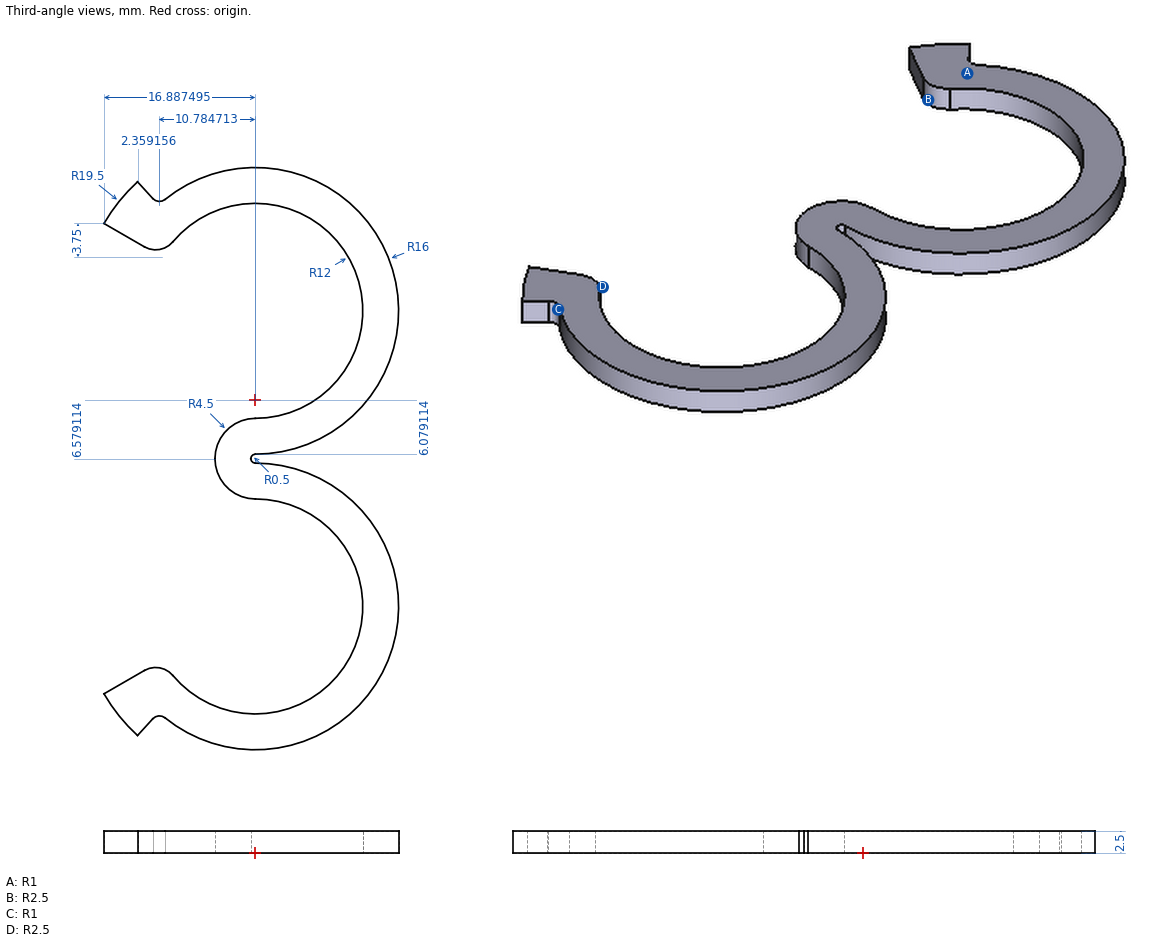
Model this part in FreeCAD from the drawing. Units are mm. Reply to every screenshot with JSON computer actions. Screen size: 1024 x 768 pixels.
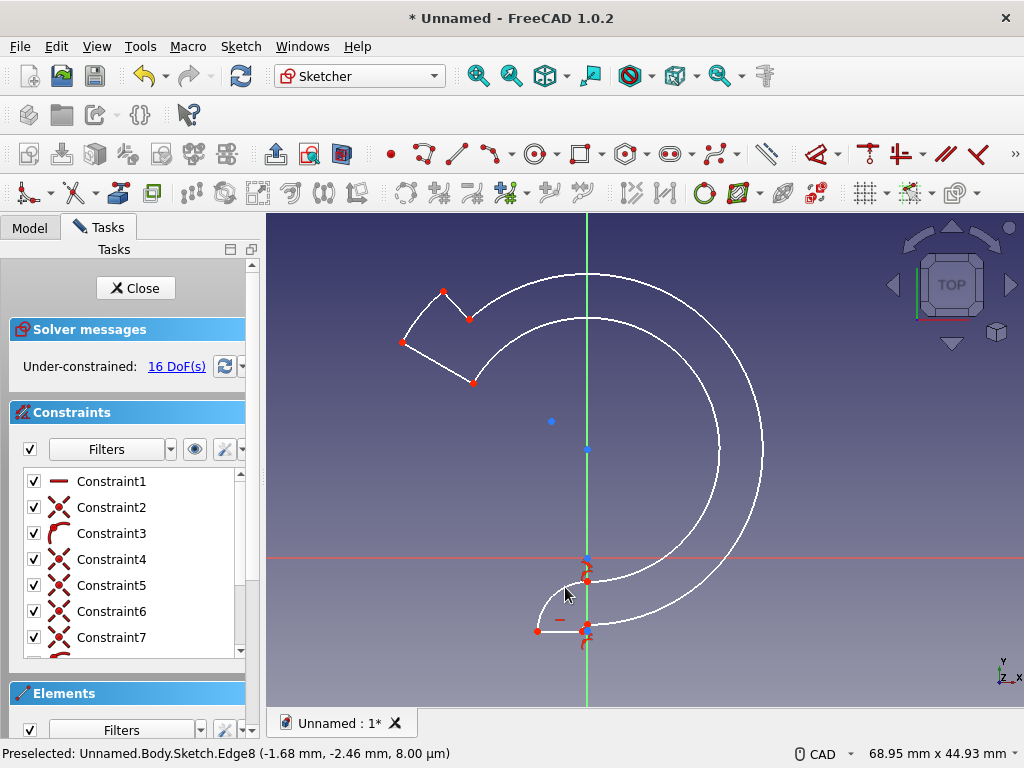
{"action": "left_click", "coordinate": [749, 519]}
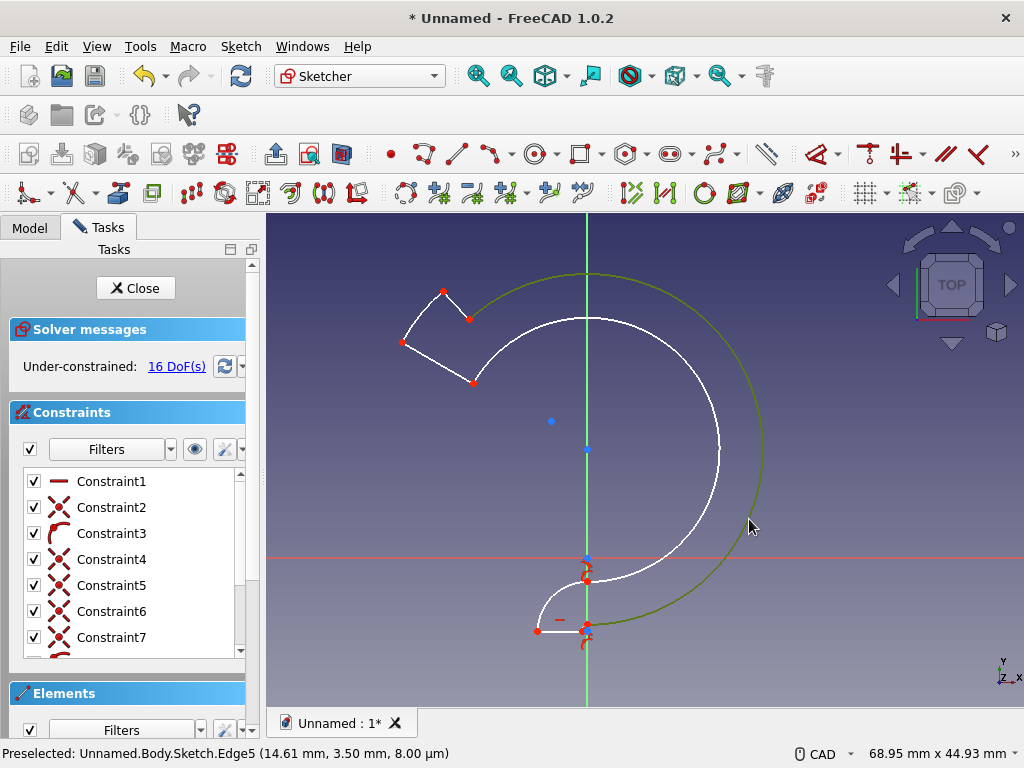
{"action": "left_click", "coordinate": [429, 305]}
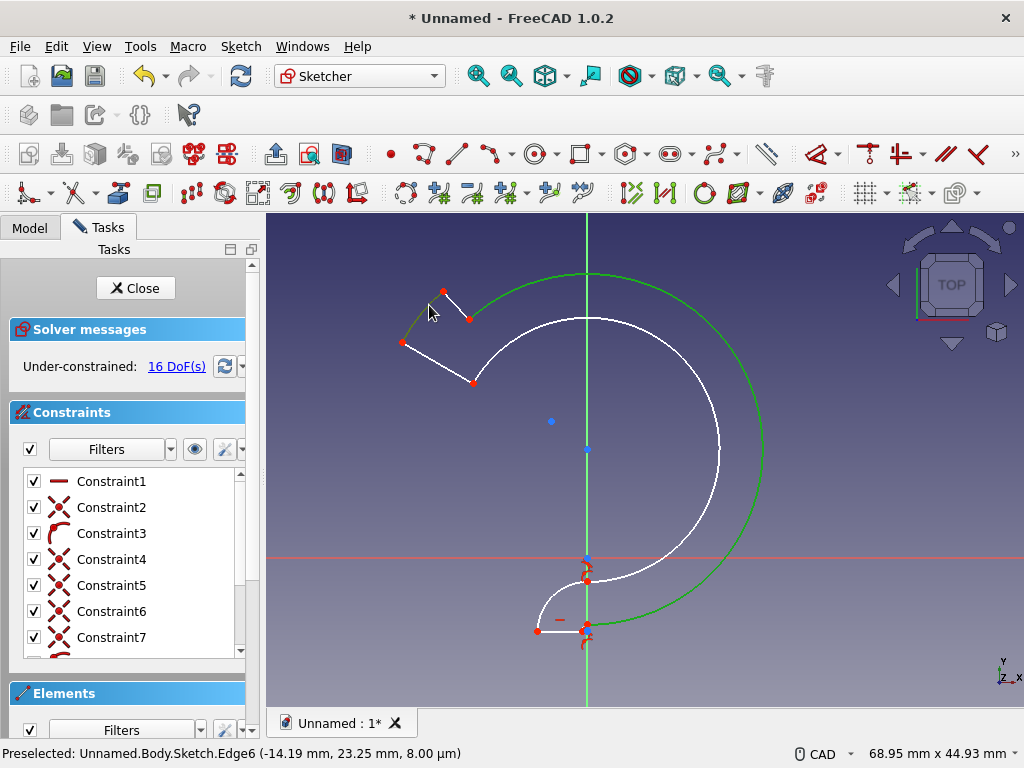
{"action": "left_click", "coordinate": [868, 154]}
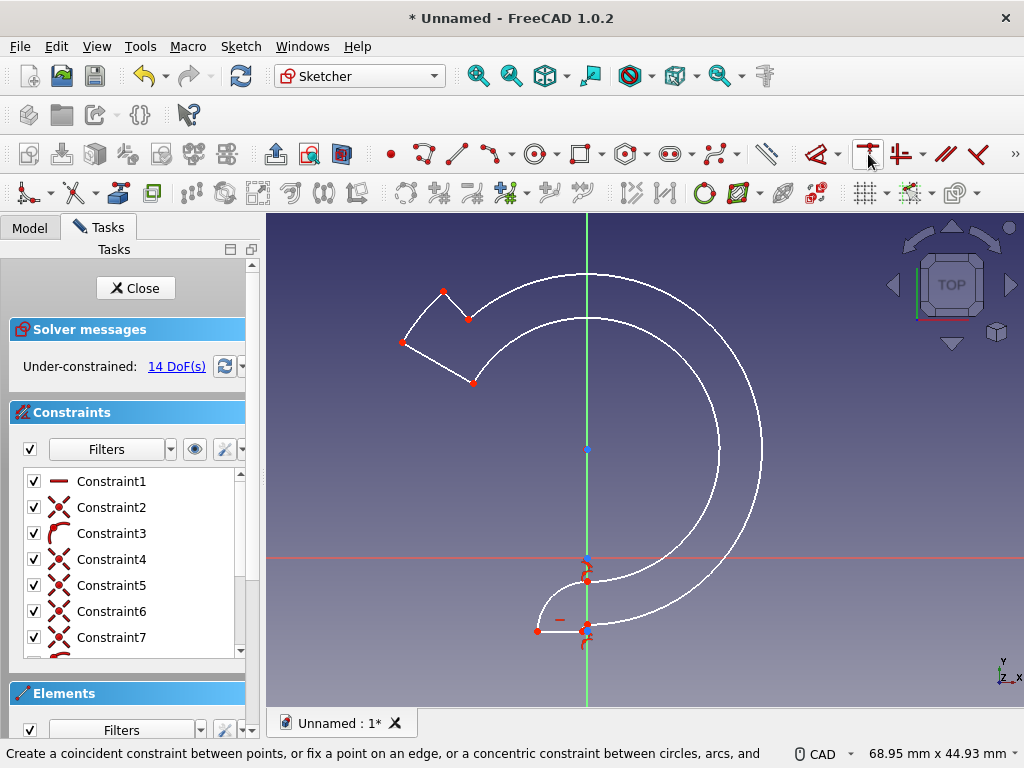
{"action": "left_click", "coordinate": [748, 518]}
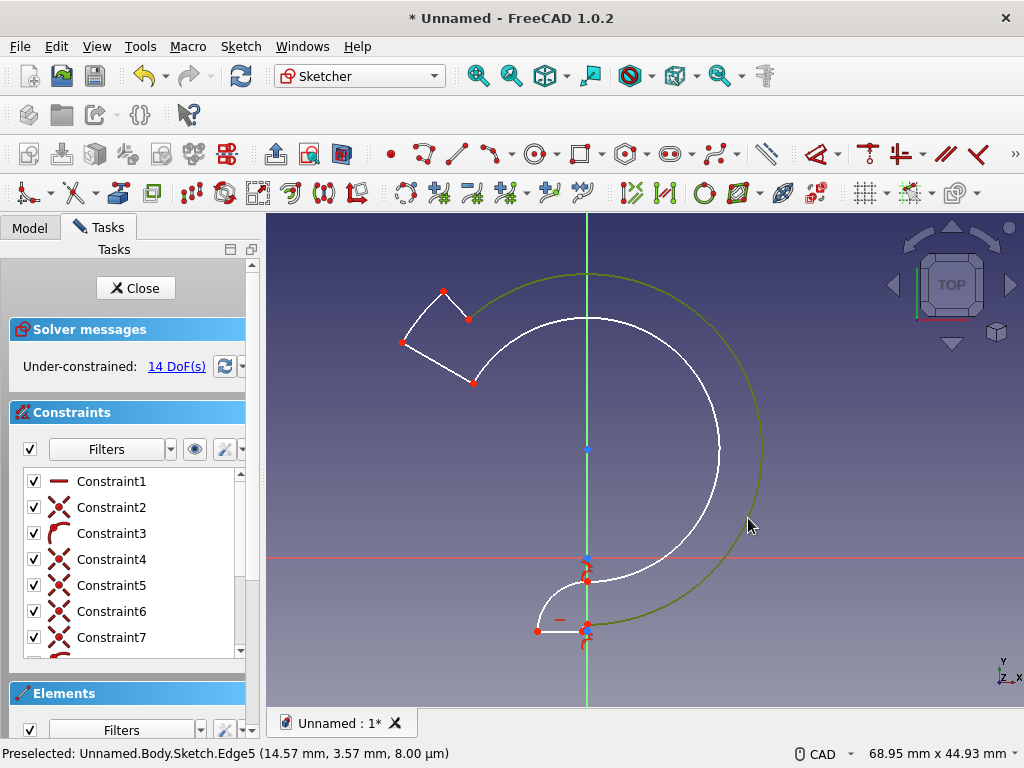
{"action": "left_click", "coordinate": [713, 491]}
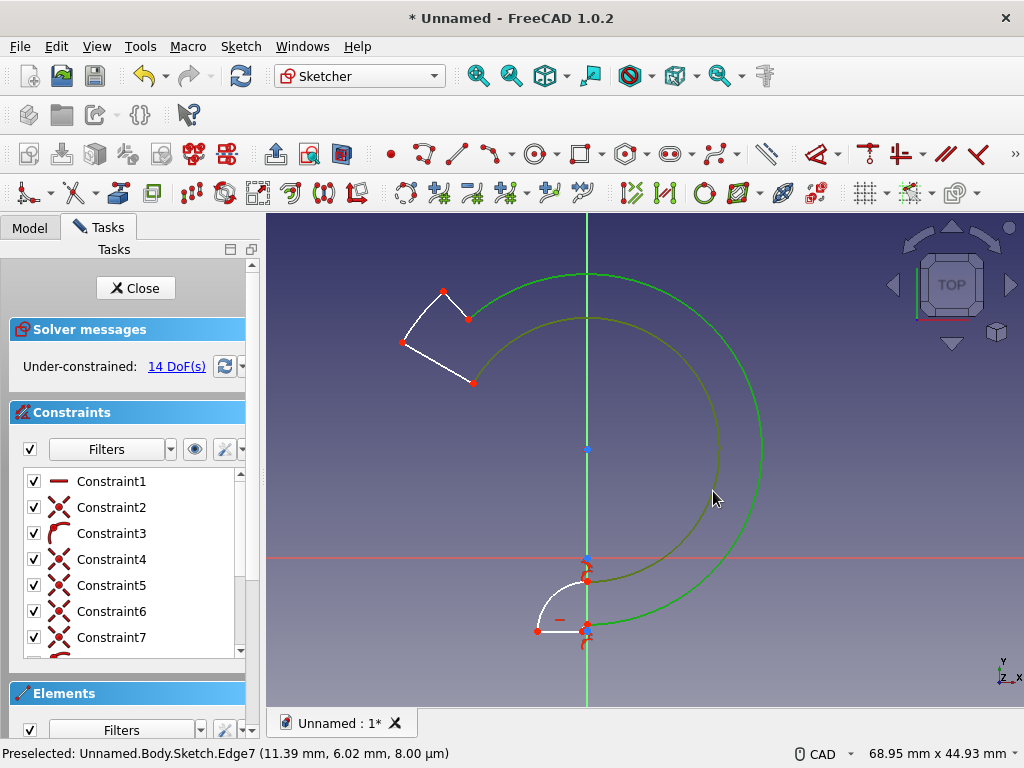
{"action": "left_click", "coordinate": [868, 154]}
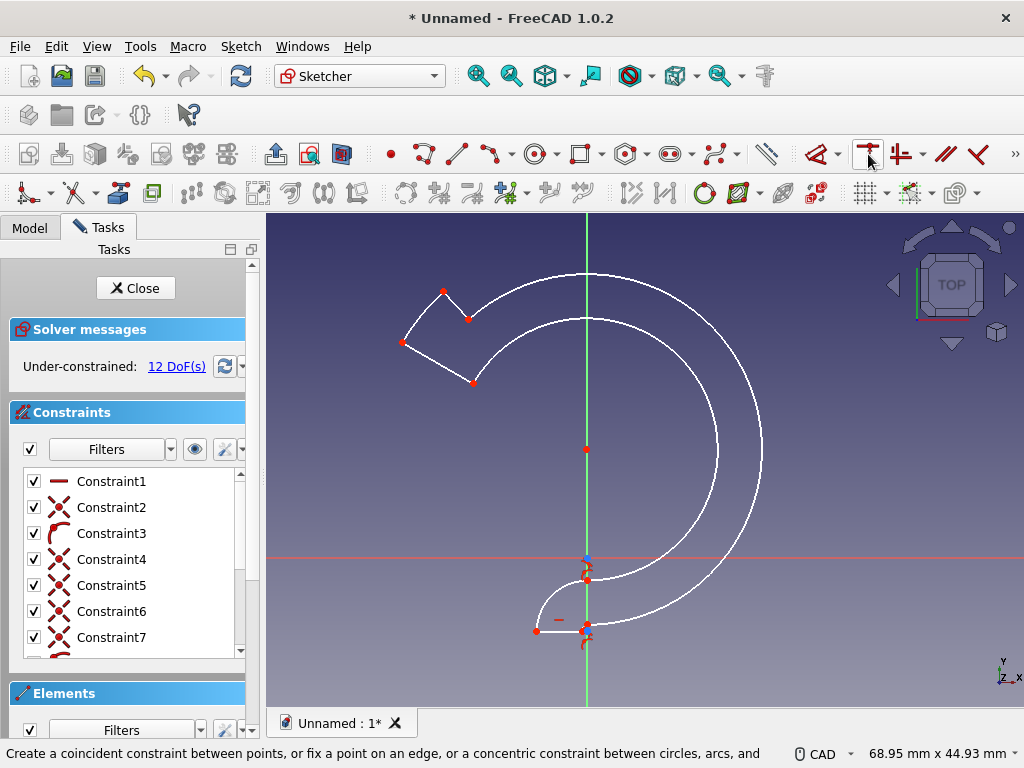
{"action": "left_click", "coordinate": [587, 449]}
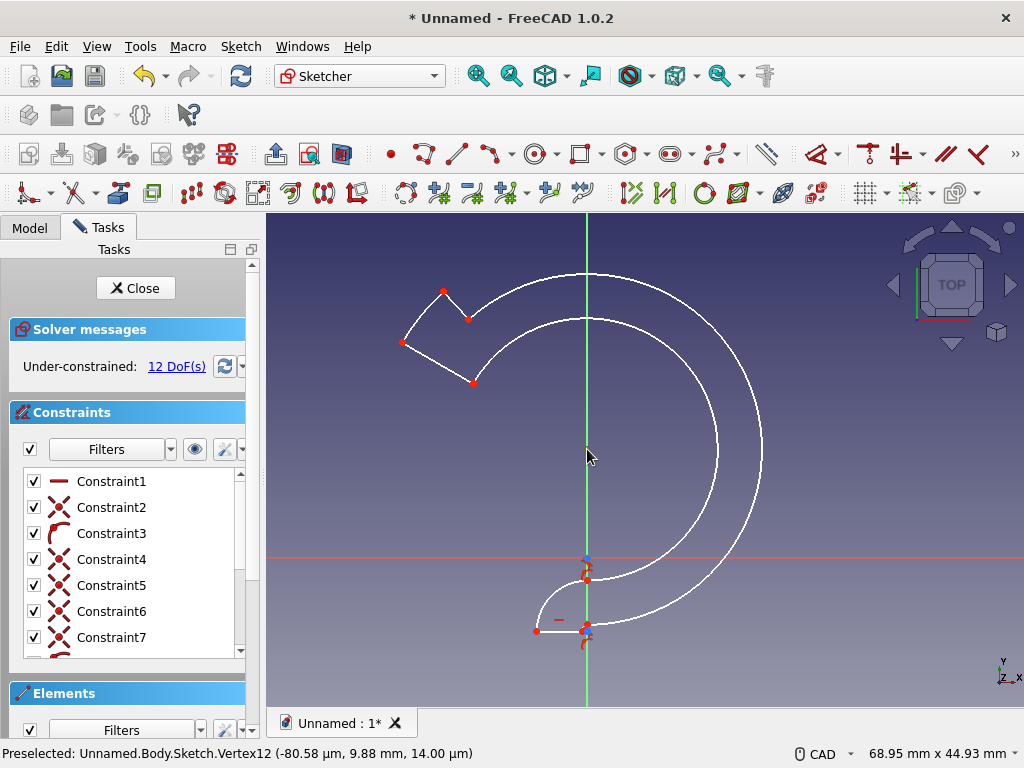
{"action": "left_click", "coordinate": [587, 523]}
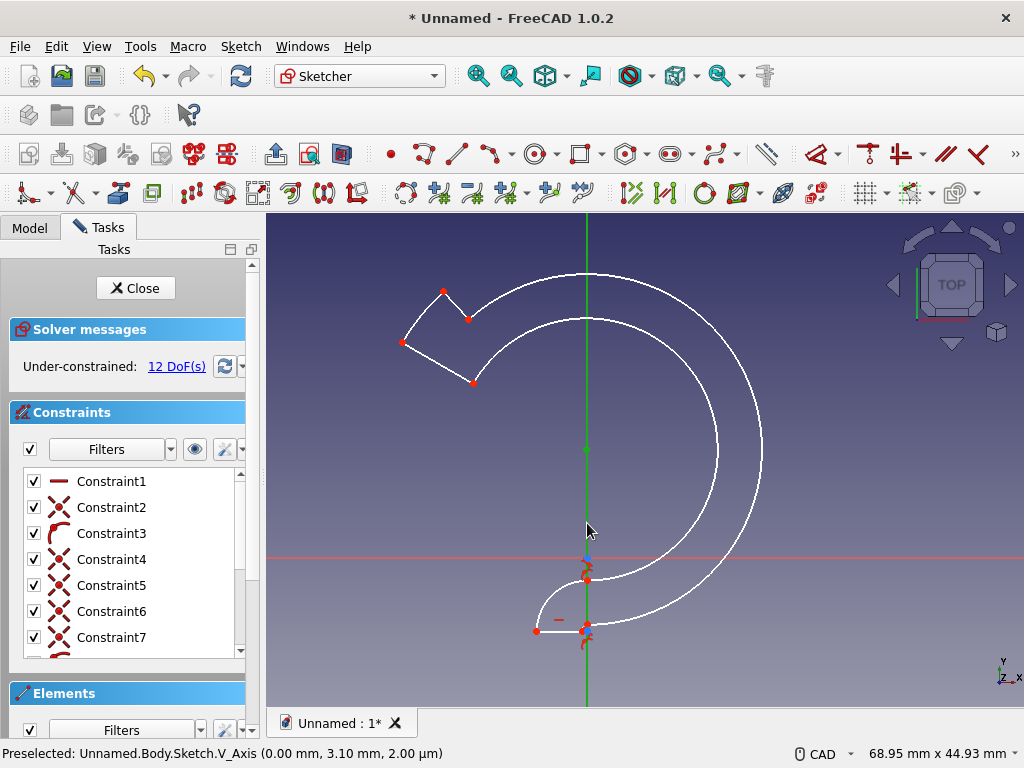
{"action": "left_click", "coordinate": [868, 154]}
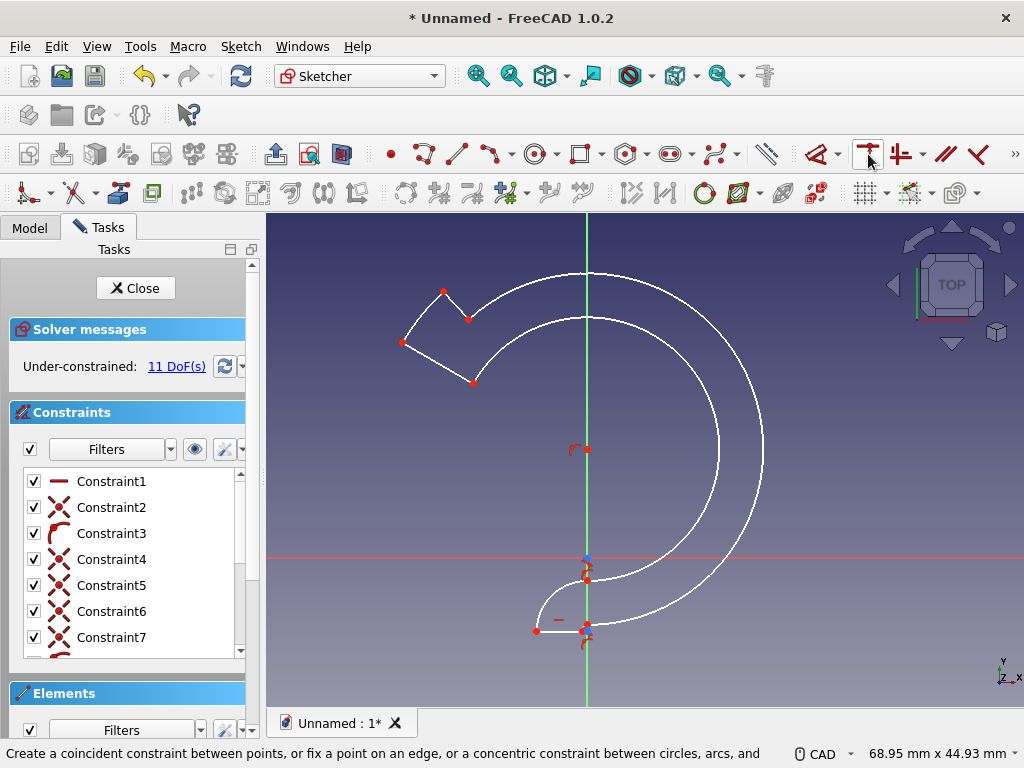
{"action": "scroll", "coordinate": [583, 627], "scroll_direction": "up", "scroll_amount": 10}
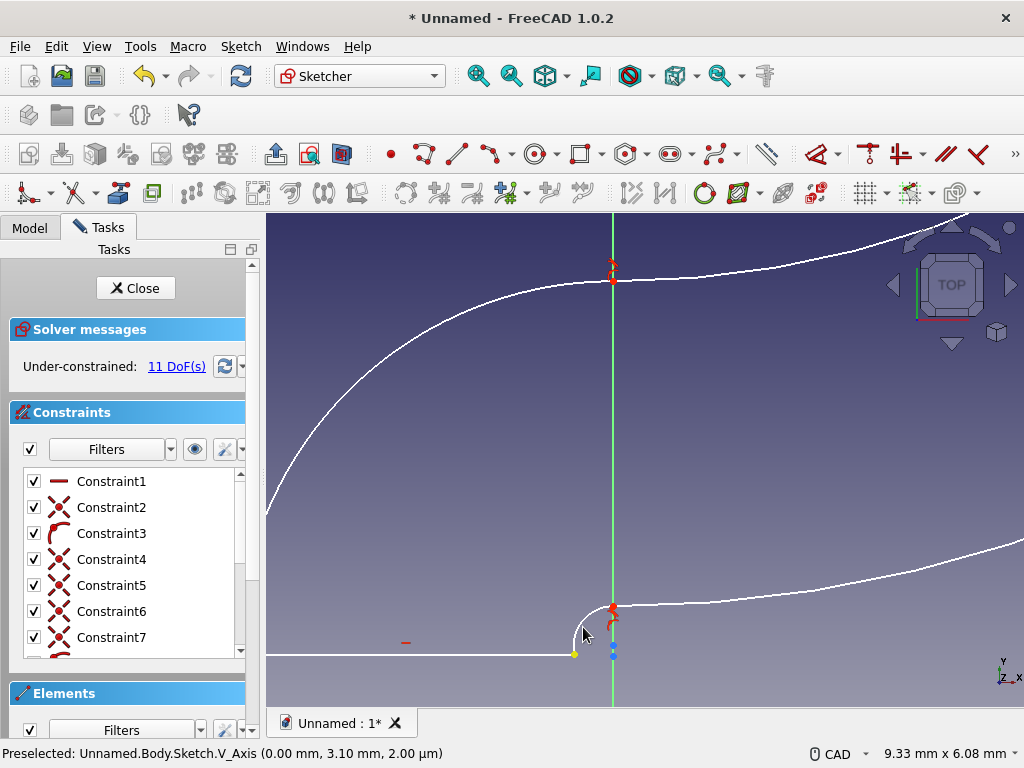
{"action": "left_click", "coordinate": [582, 621]}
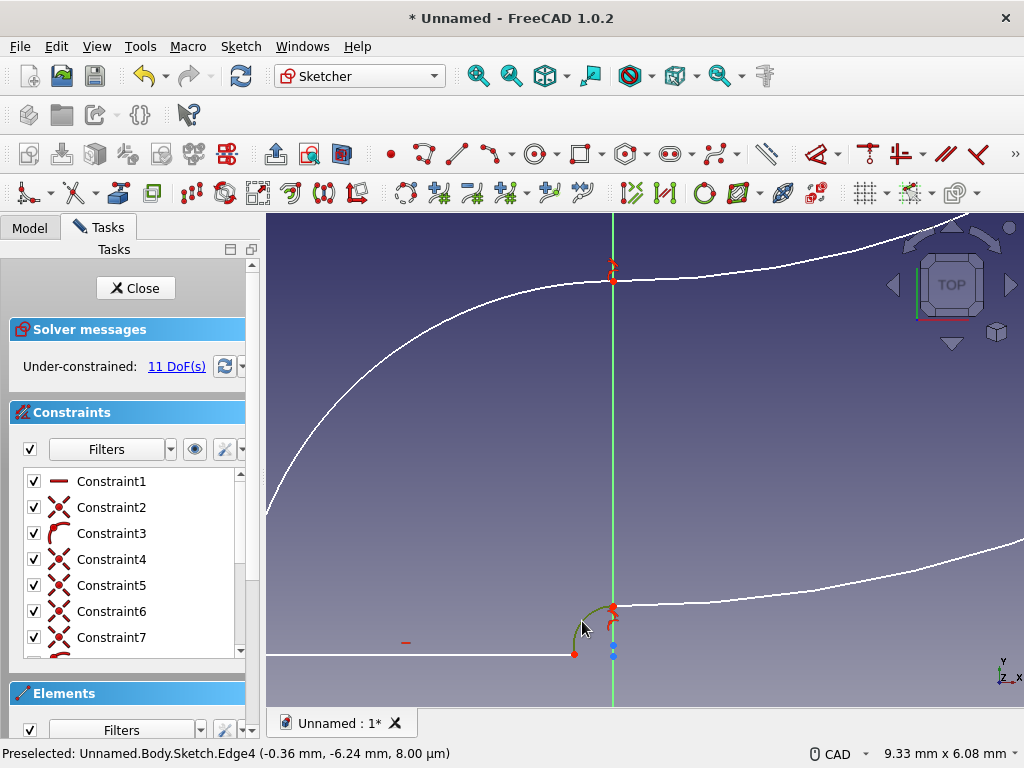
{"action": "left_click", "coordinate": [838, 154]}